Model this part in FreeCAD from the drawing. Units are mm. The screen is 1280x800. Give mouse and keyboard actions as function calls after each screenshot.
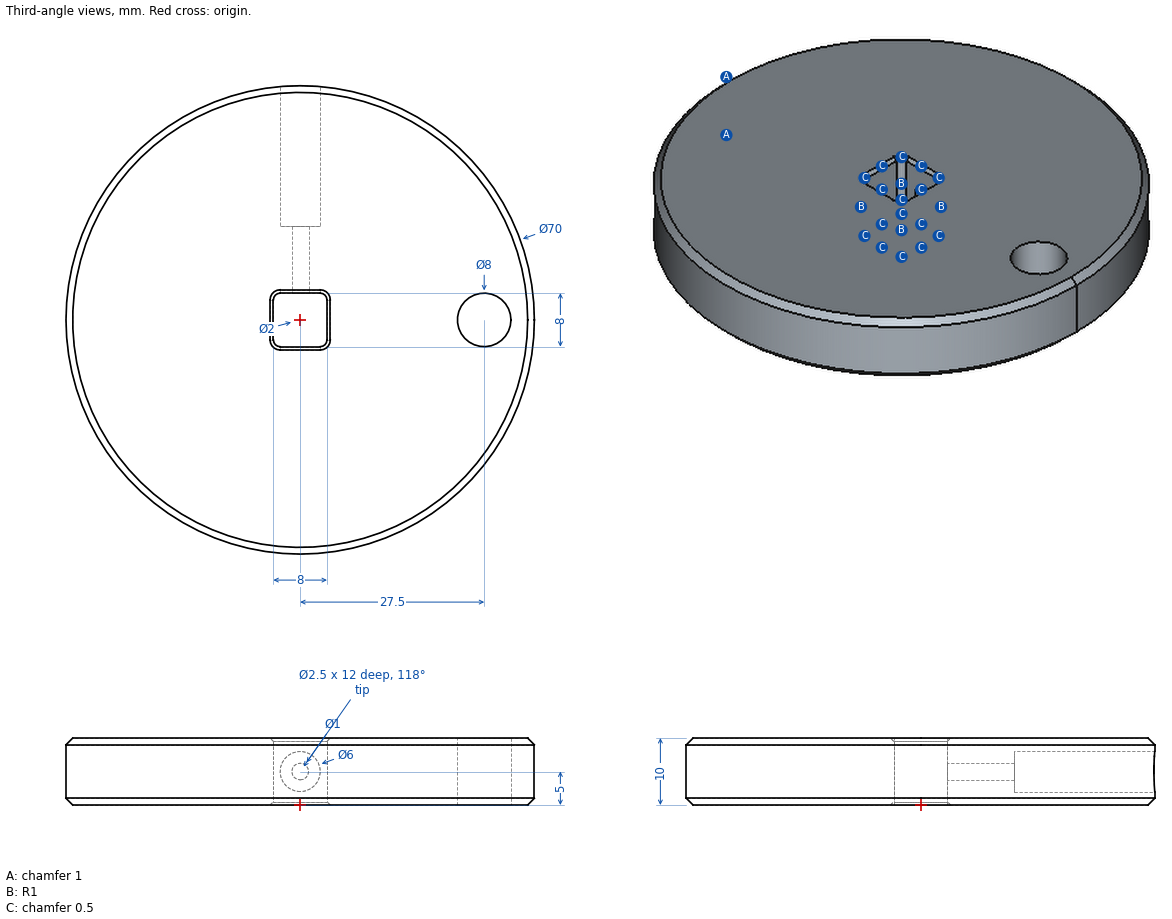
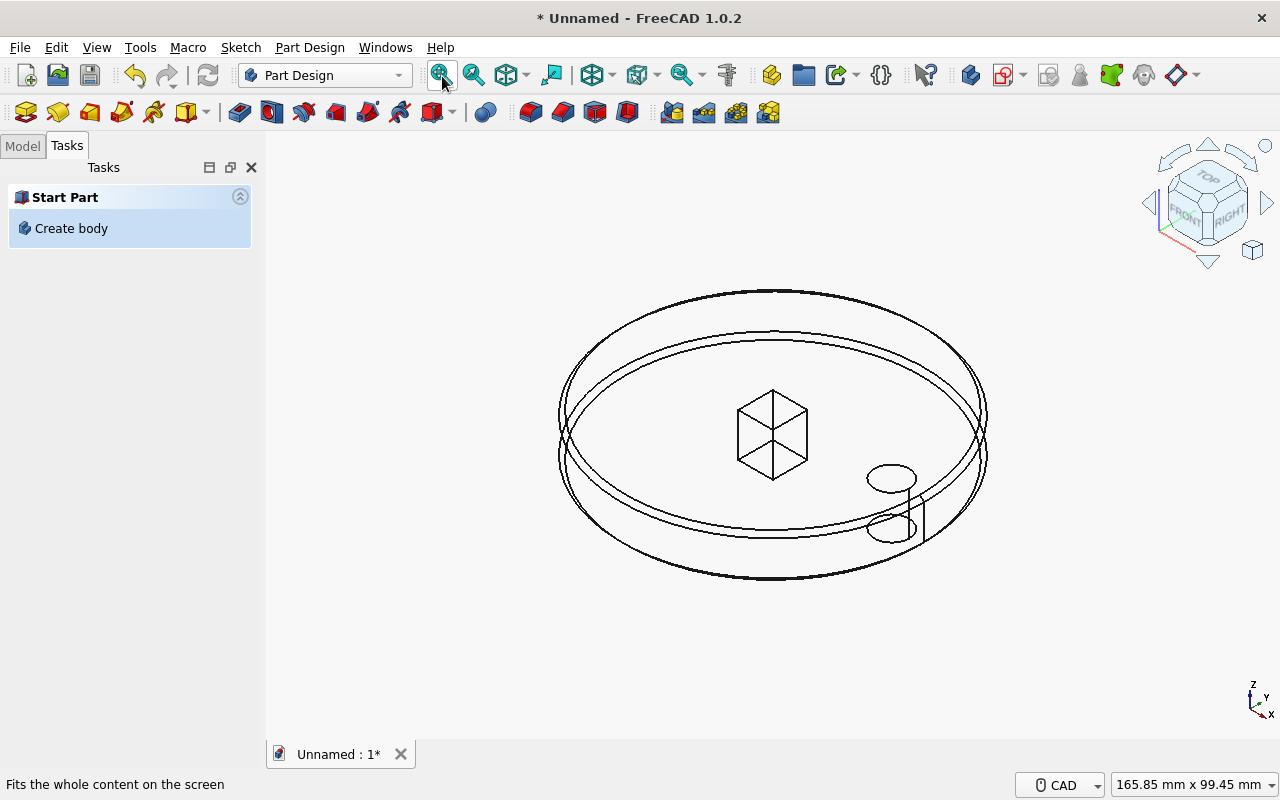
click(807, 434)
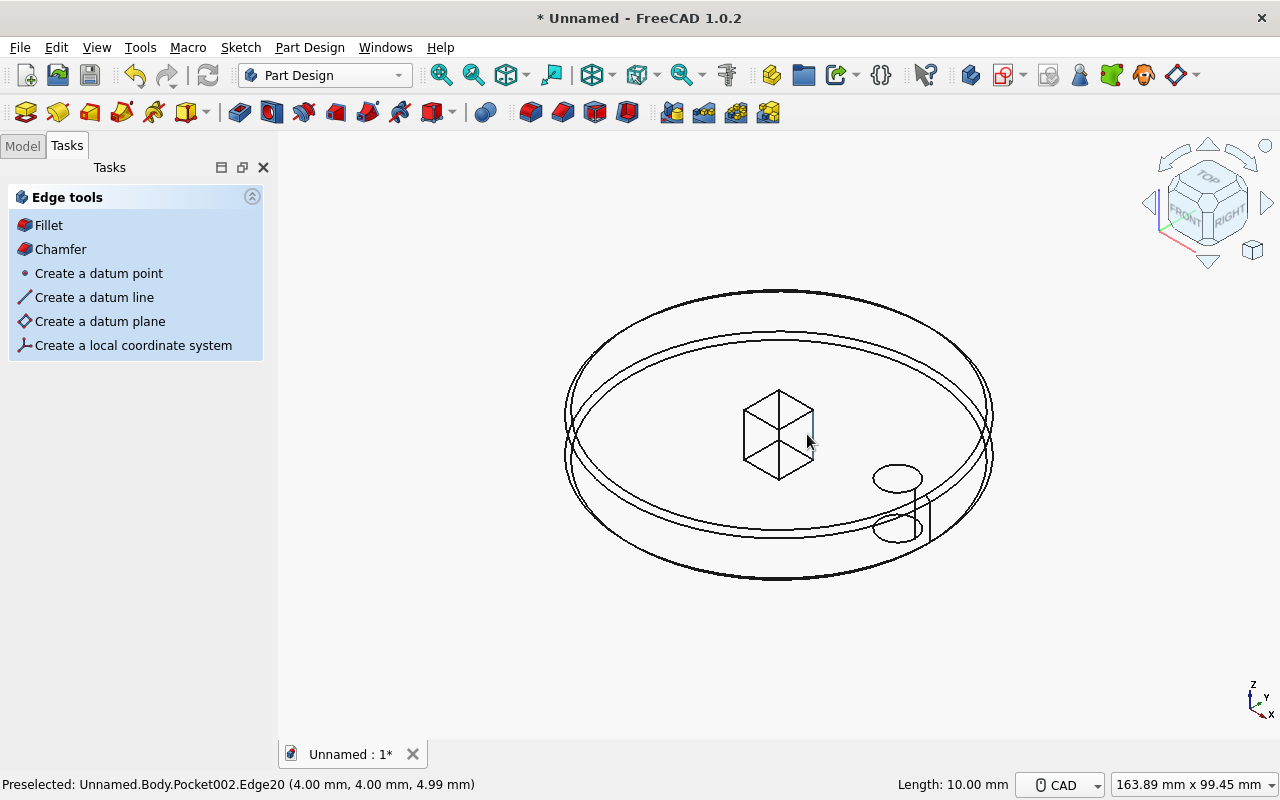
click(779, 454, ctrl)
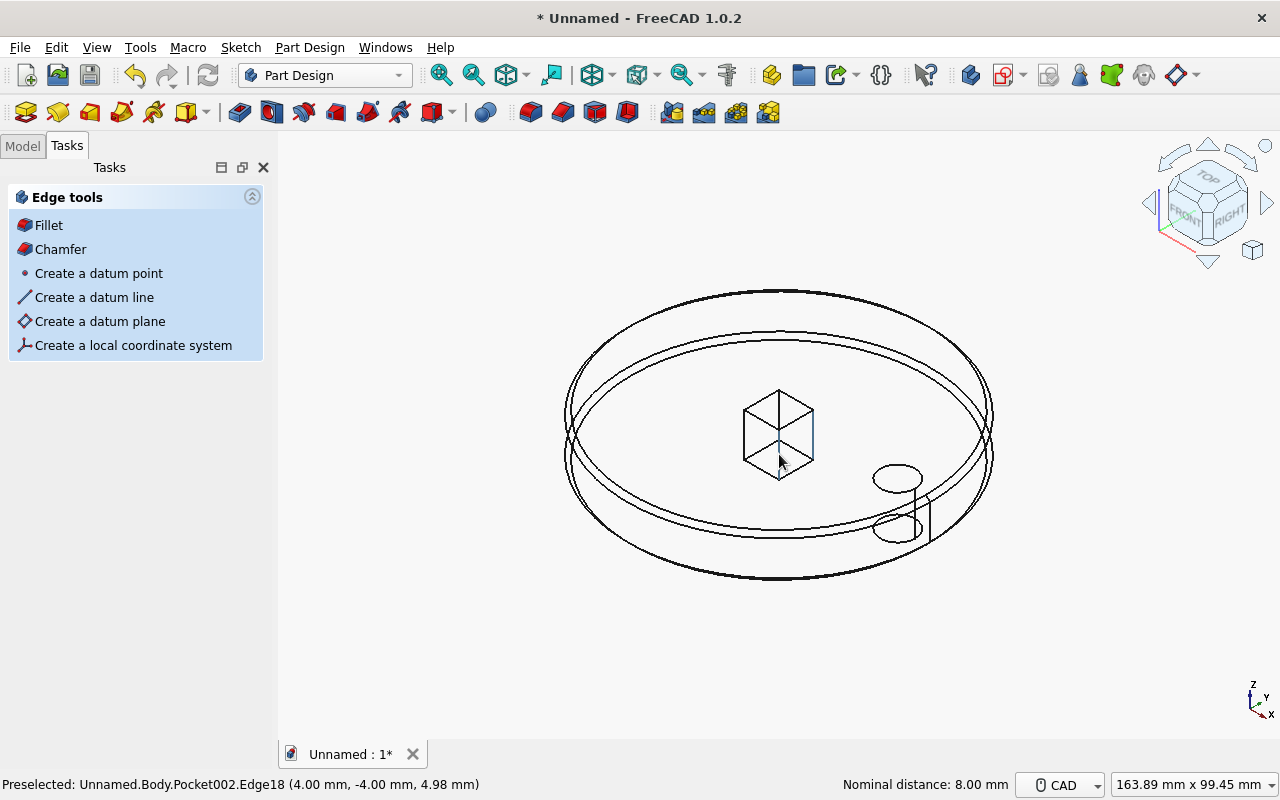
click(744, 434, ctrl)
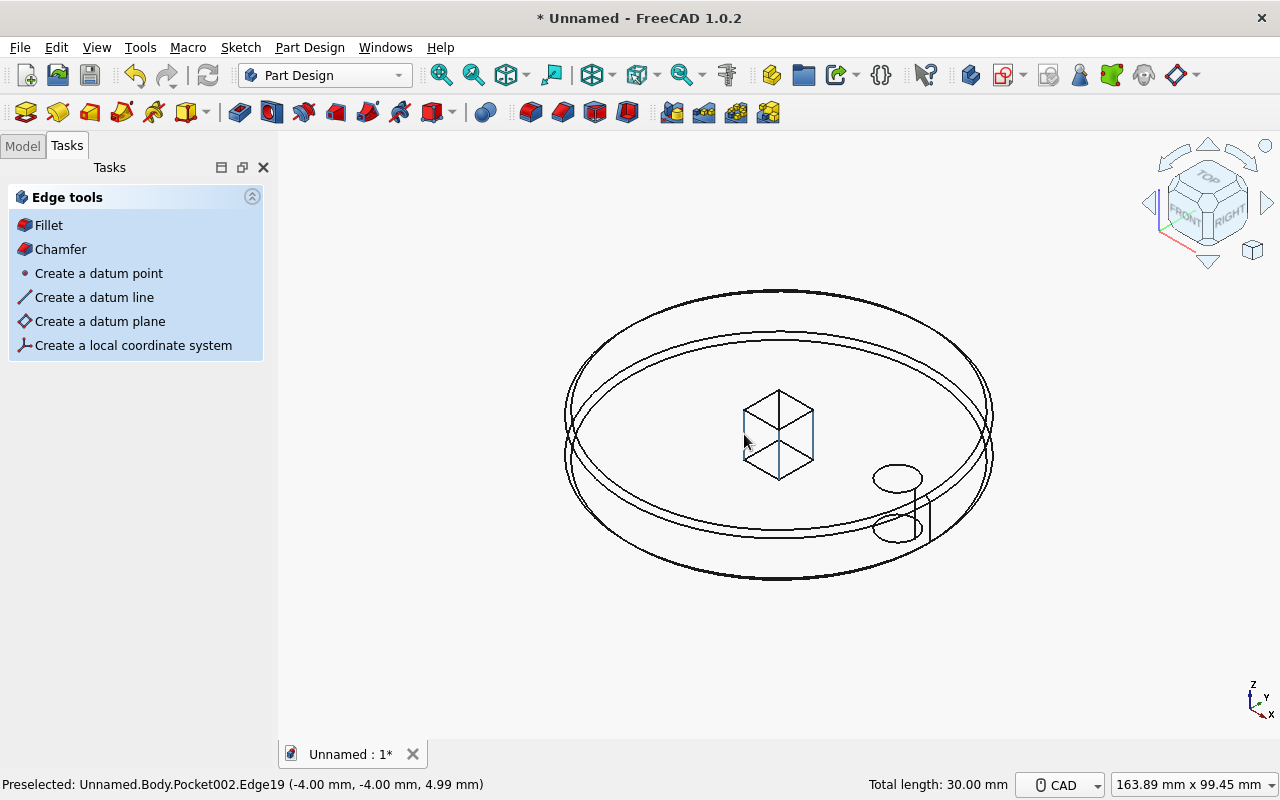
click(779, 414, ctrl)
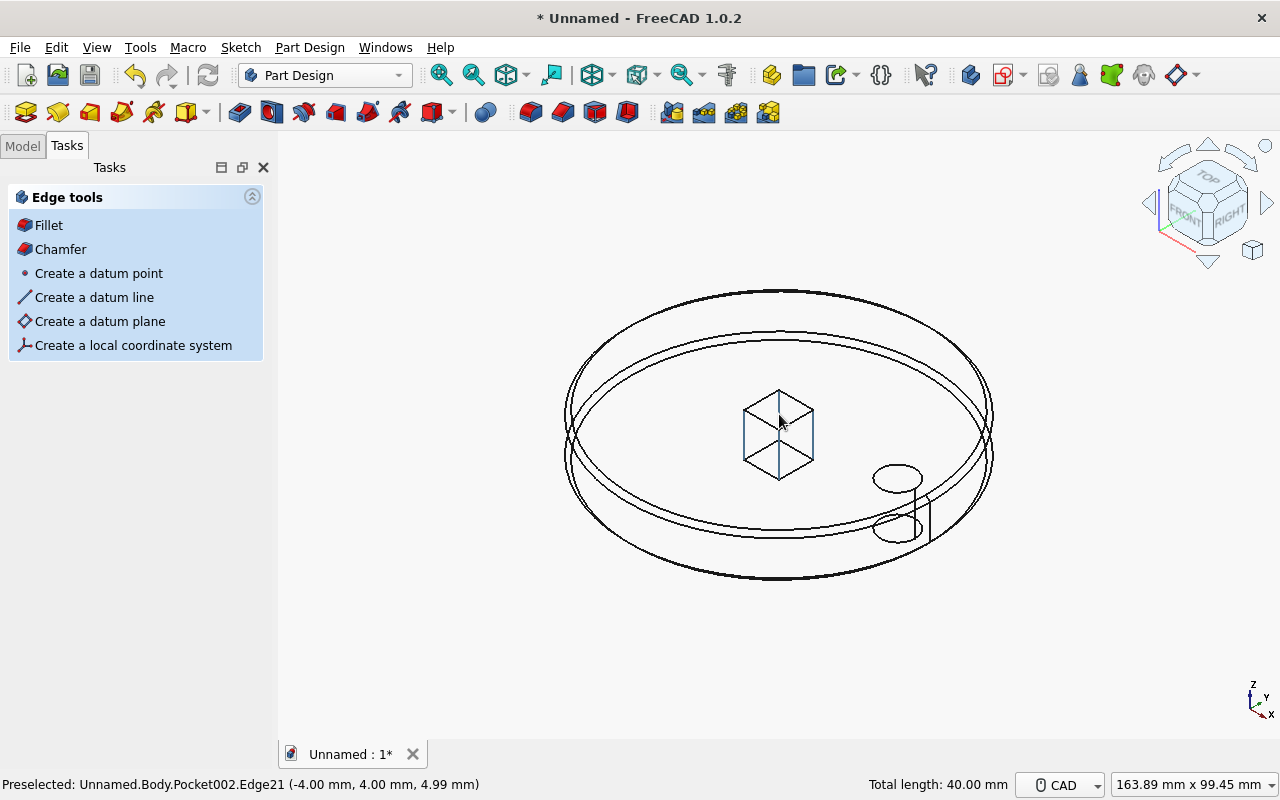
key(v)
key(1)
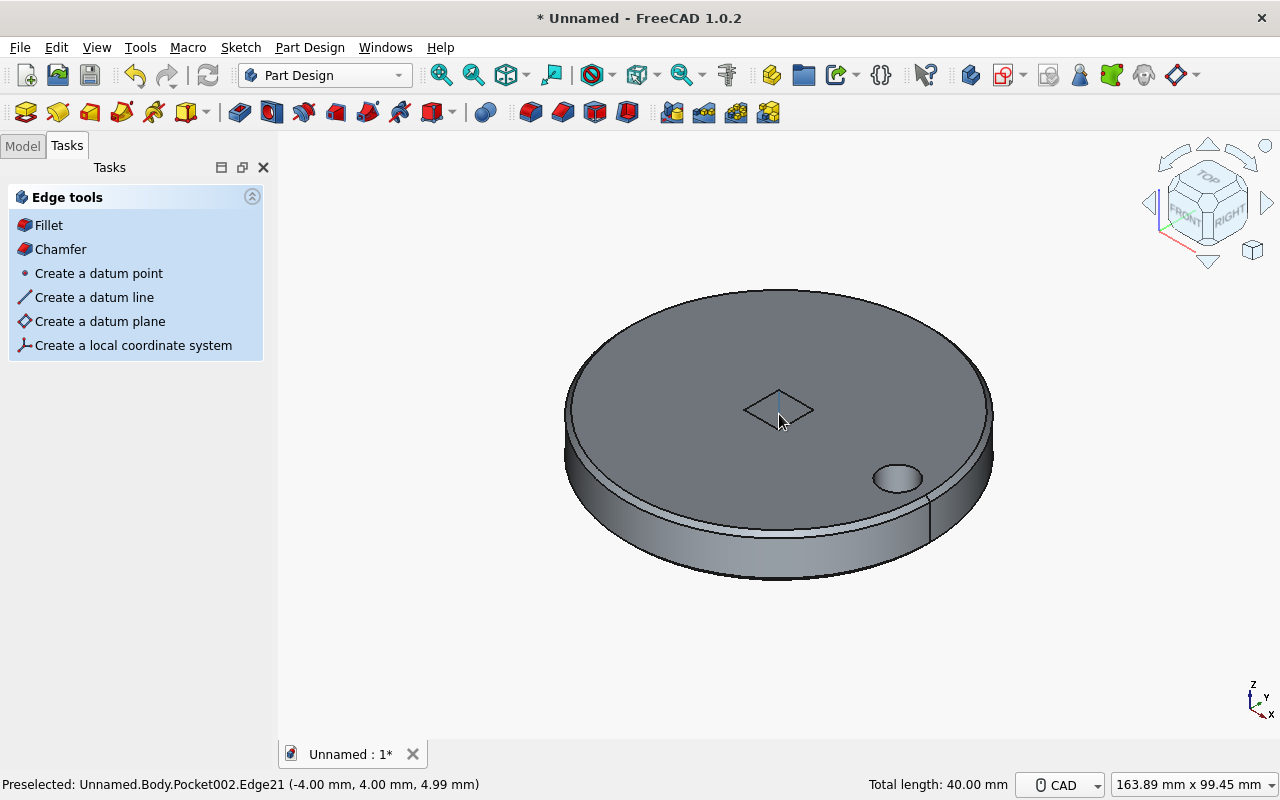
click(532, 112)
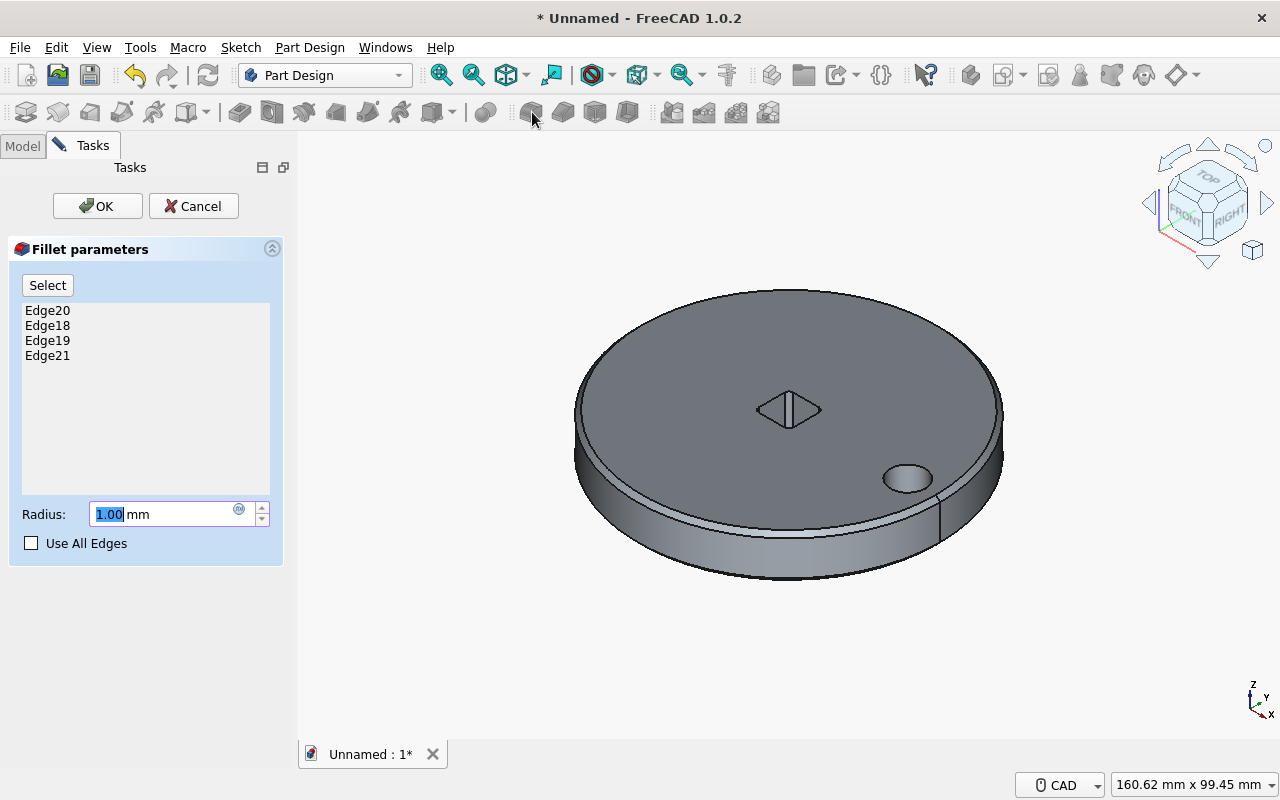
text(1)
key(Tab)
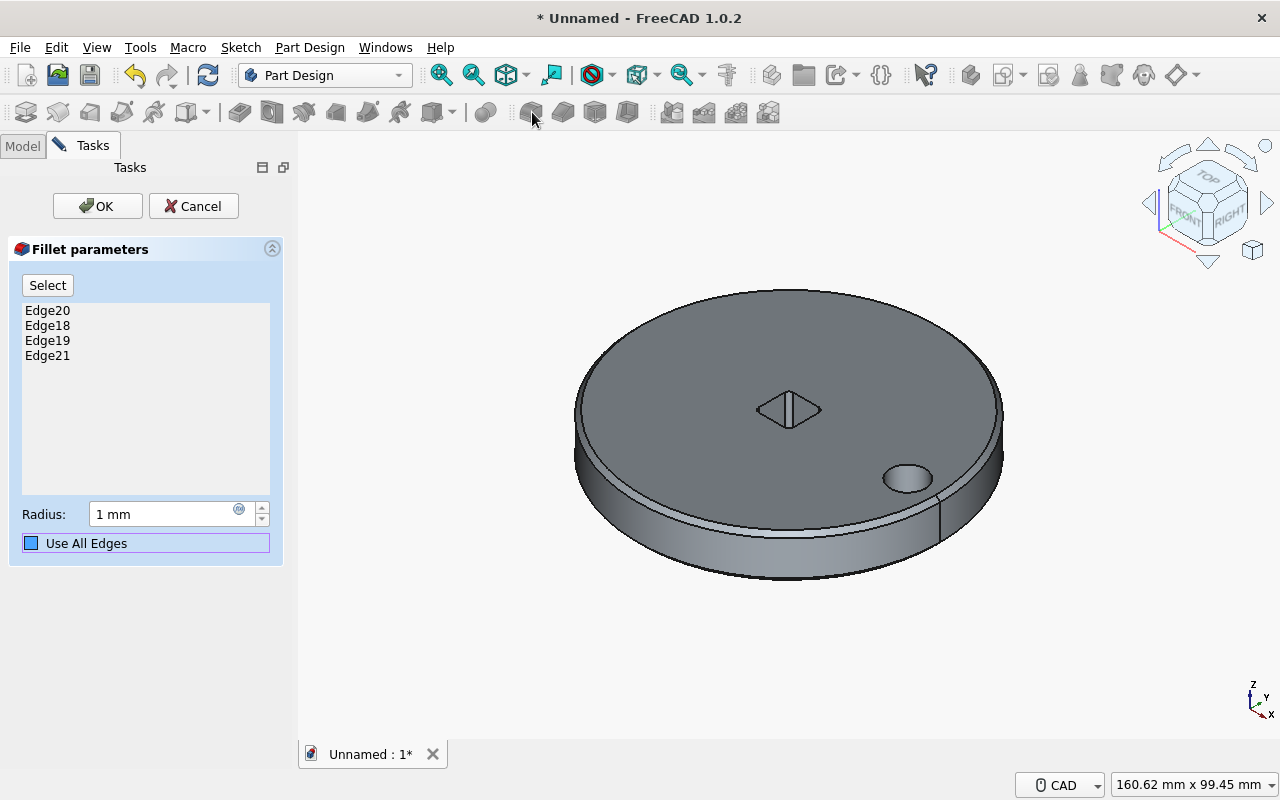
click(98, 206)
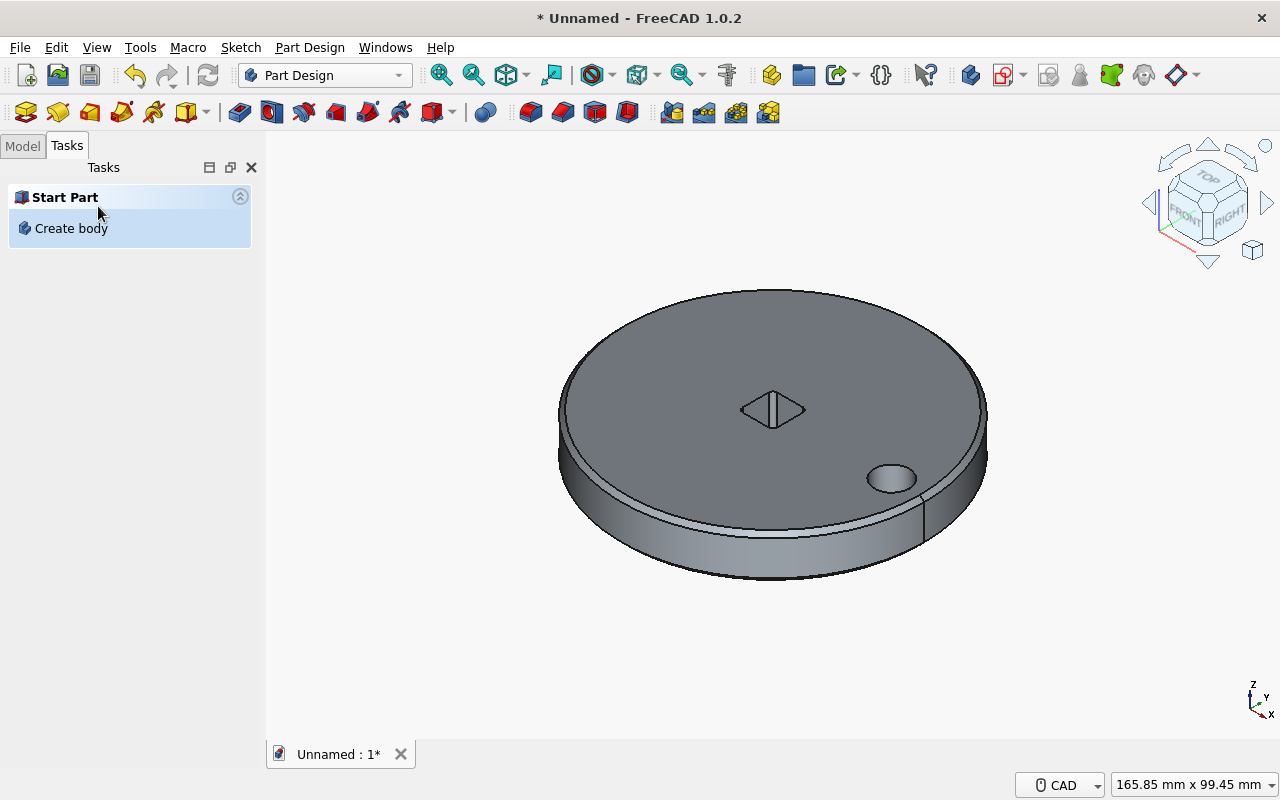
click(23, 145)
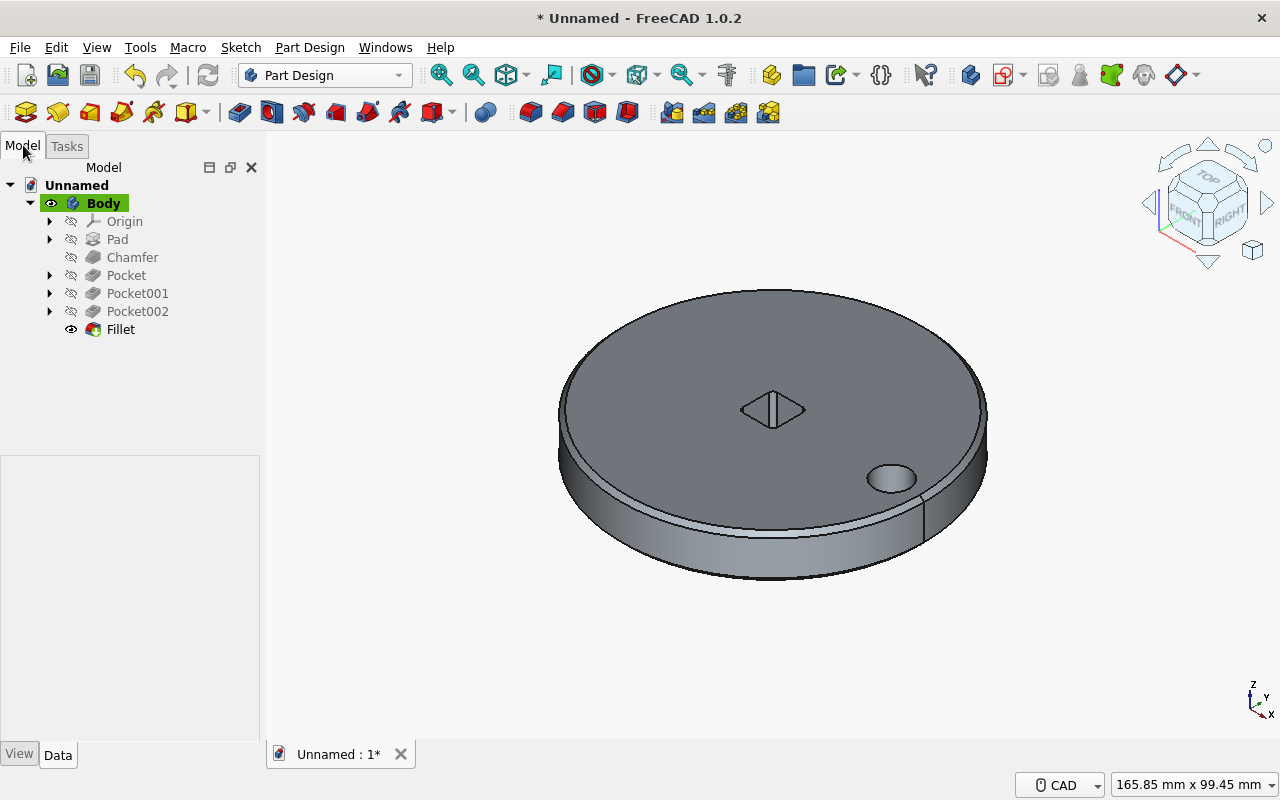
click(50, 221)